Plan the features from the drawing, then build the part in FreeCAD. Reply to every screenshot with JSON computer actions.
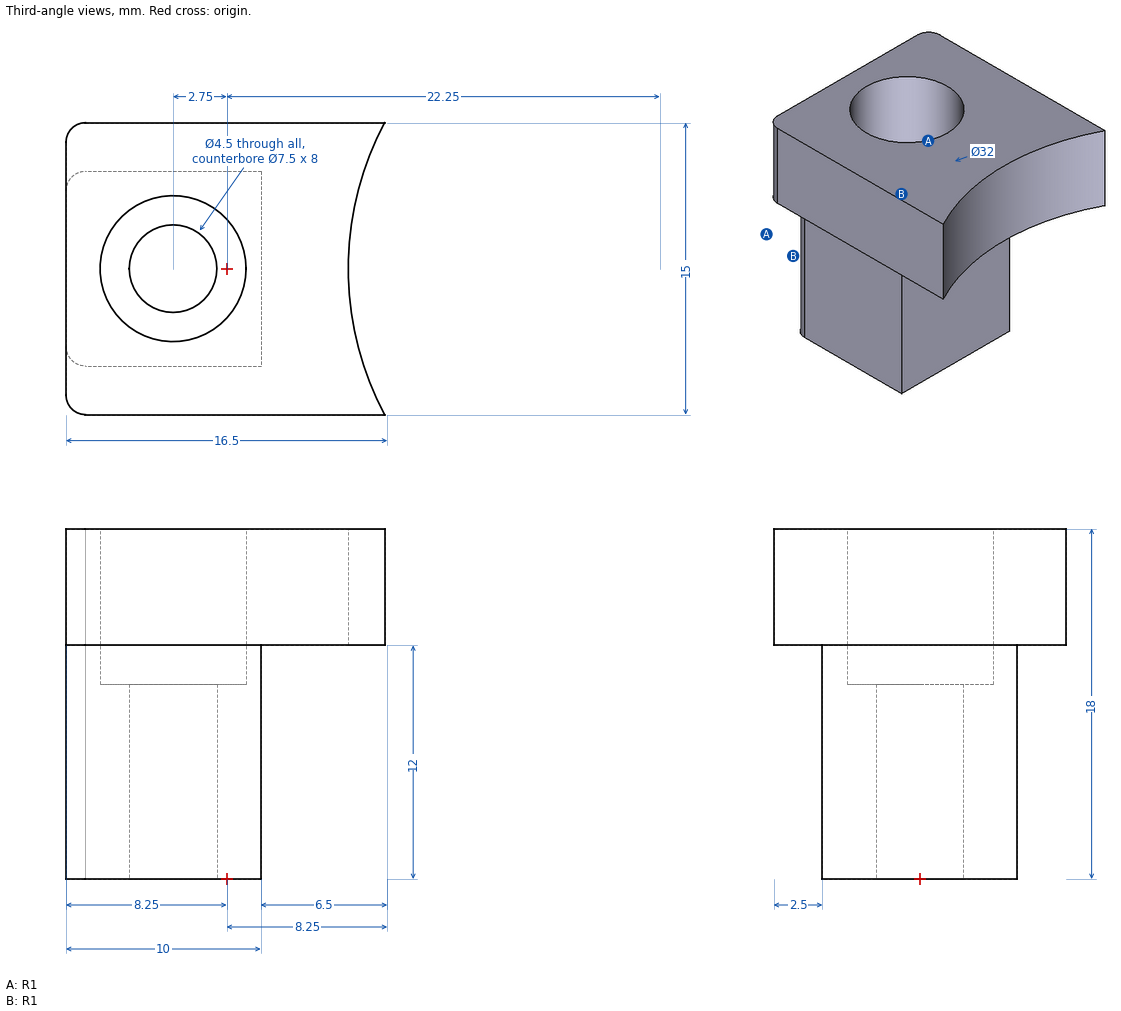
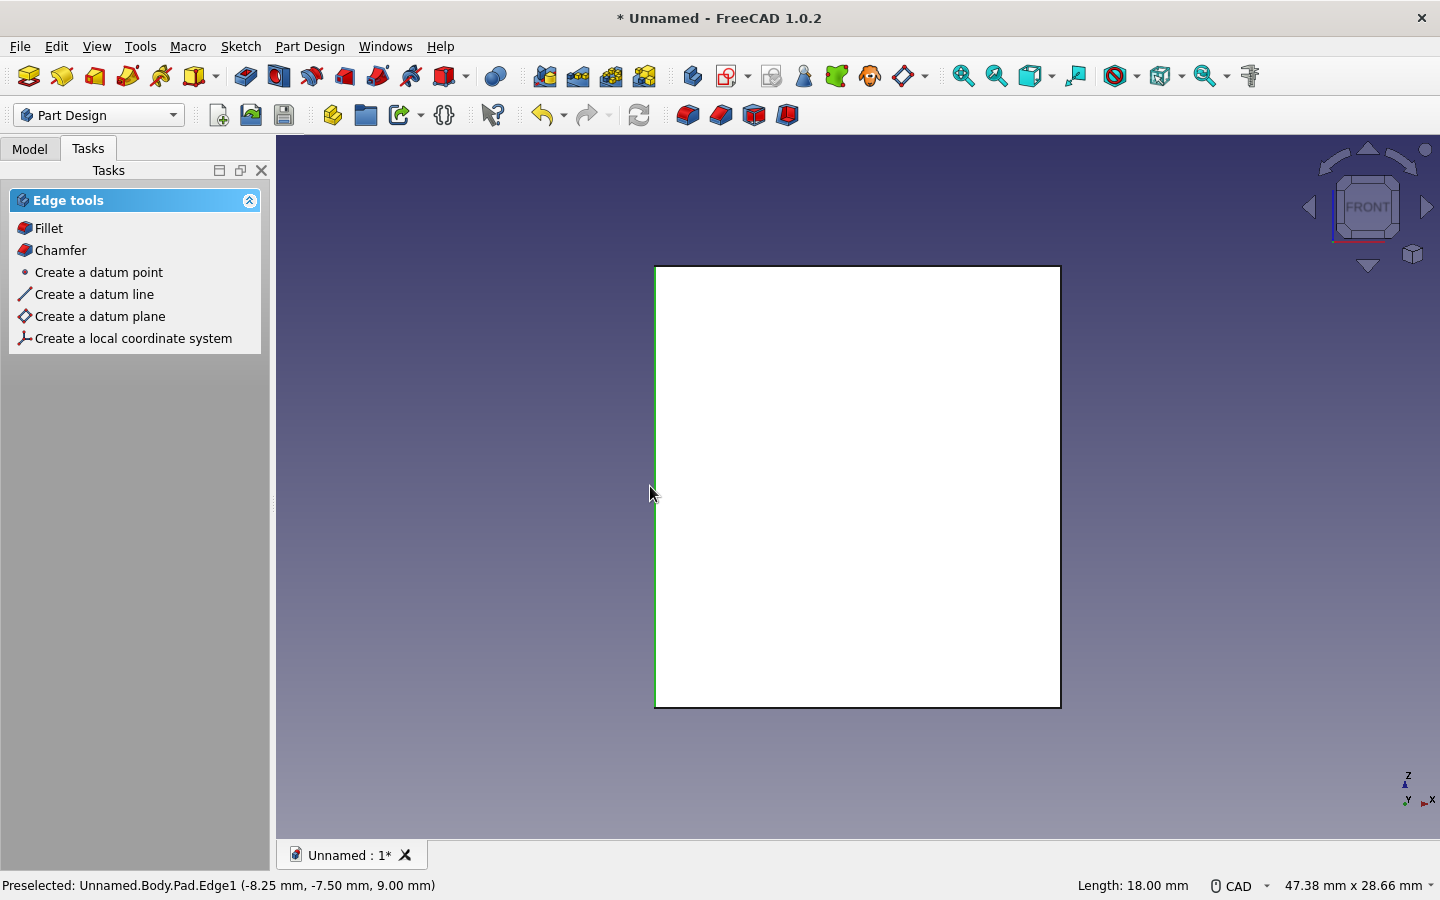
{"action": "key", "text": "3"}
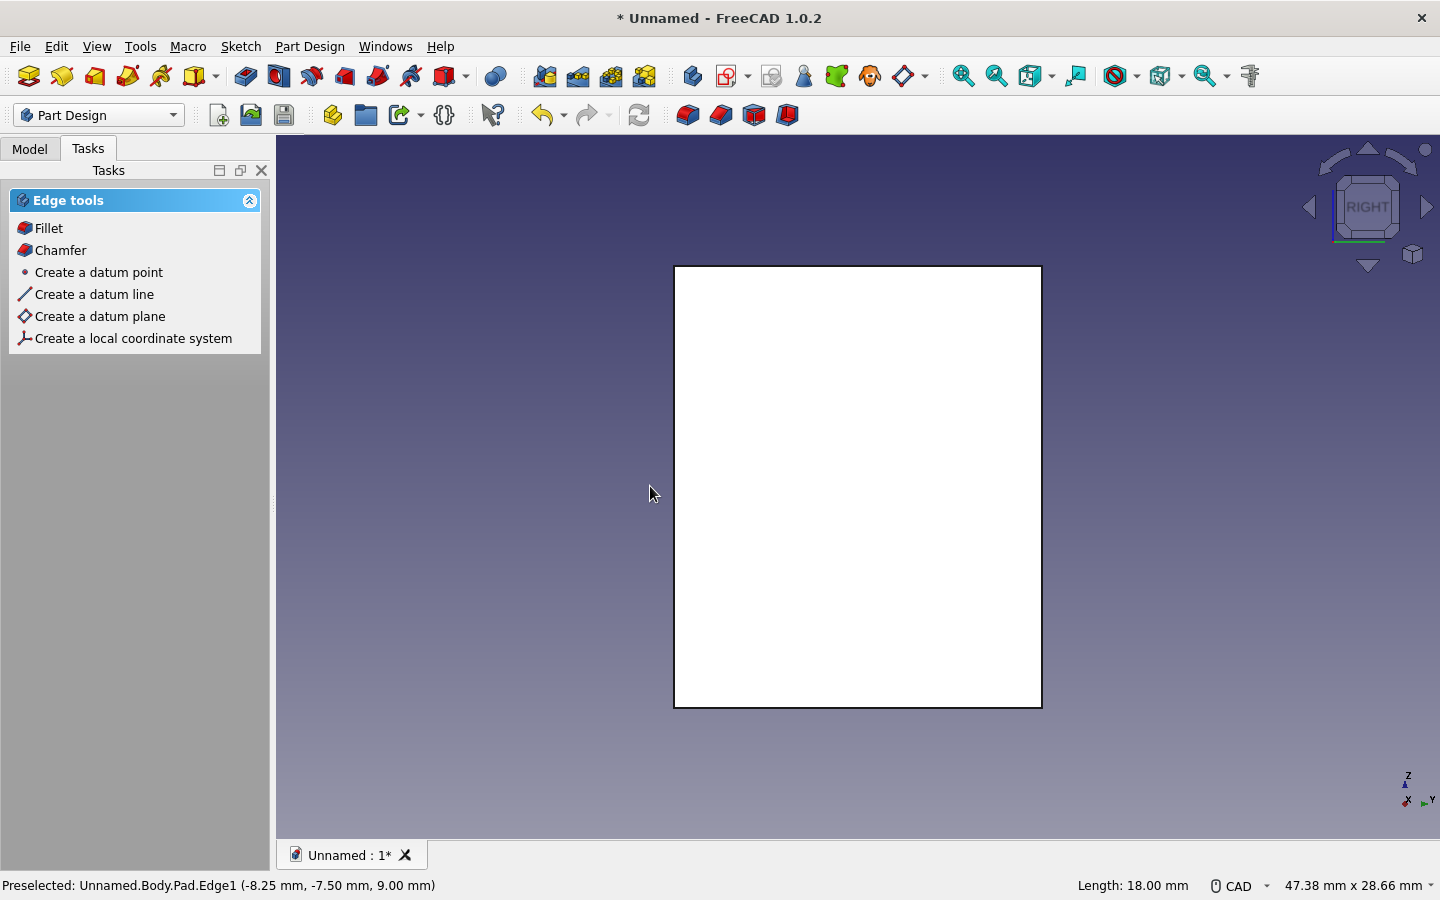
{"action": "key", "text": "5"}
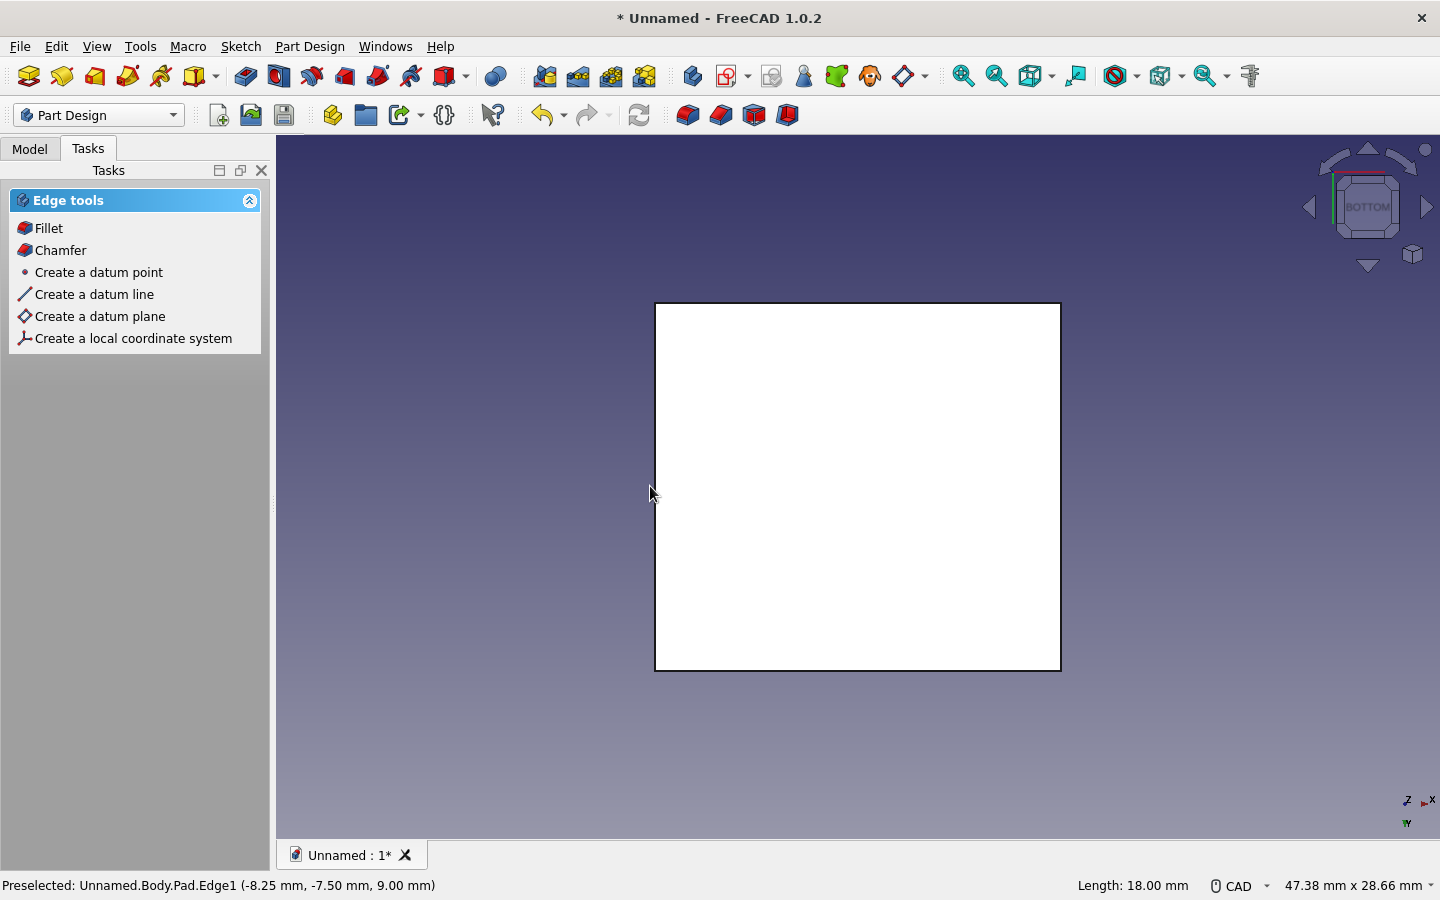
{"action": "key", "text": "4"}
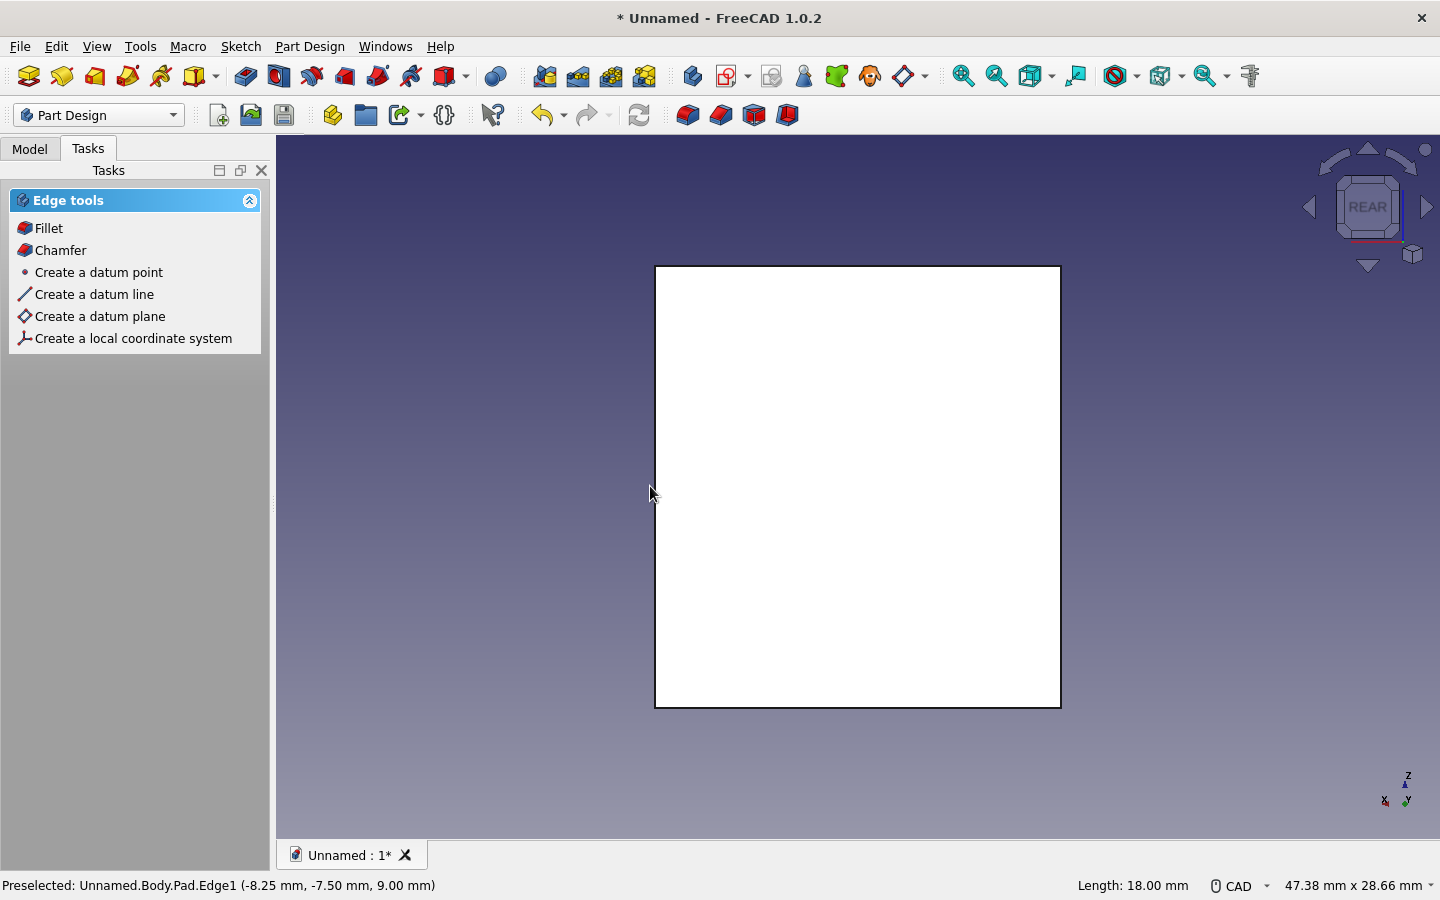
{"action": "left_click", "coordinate": [1061, 486], "text": "ctrl"}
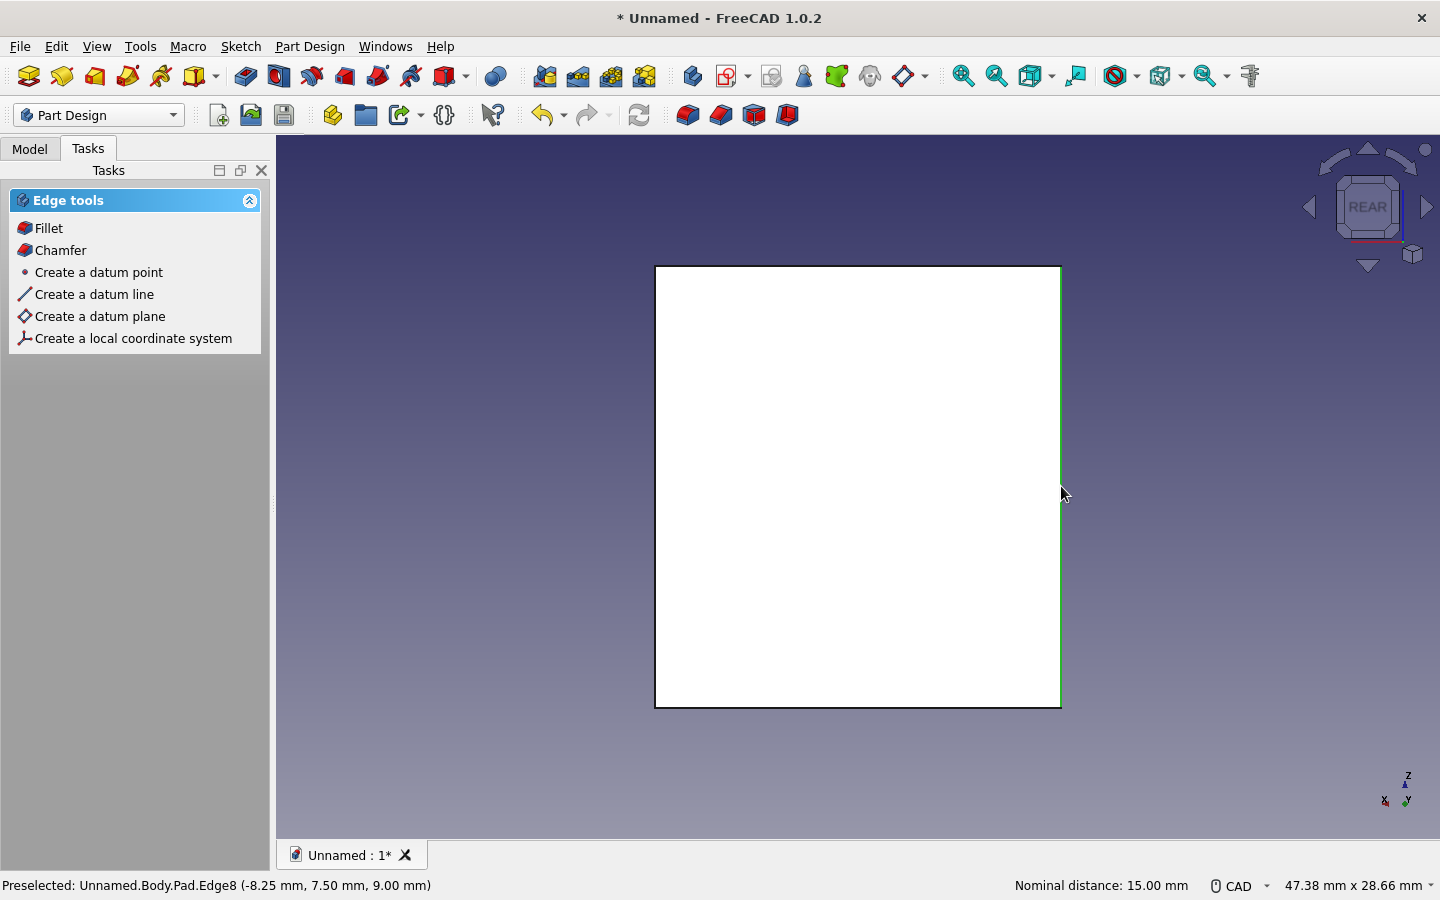
{"action": "left_click", "coordinate": [688, 116]}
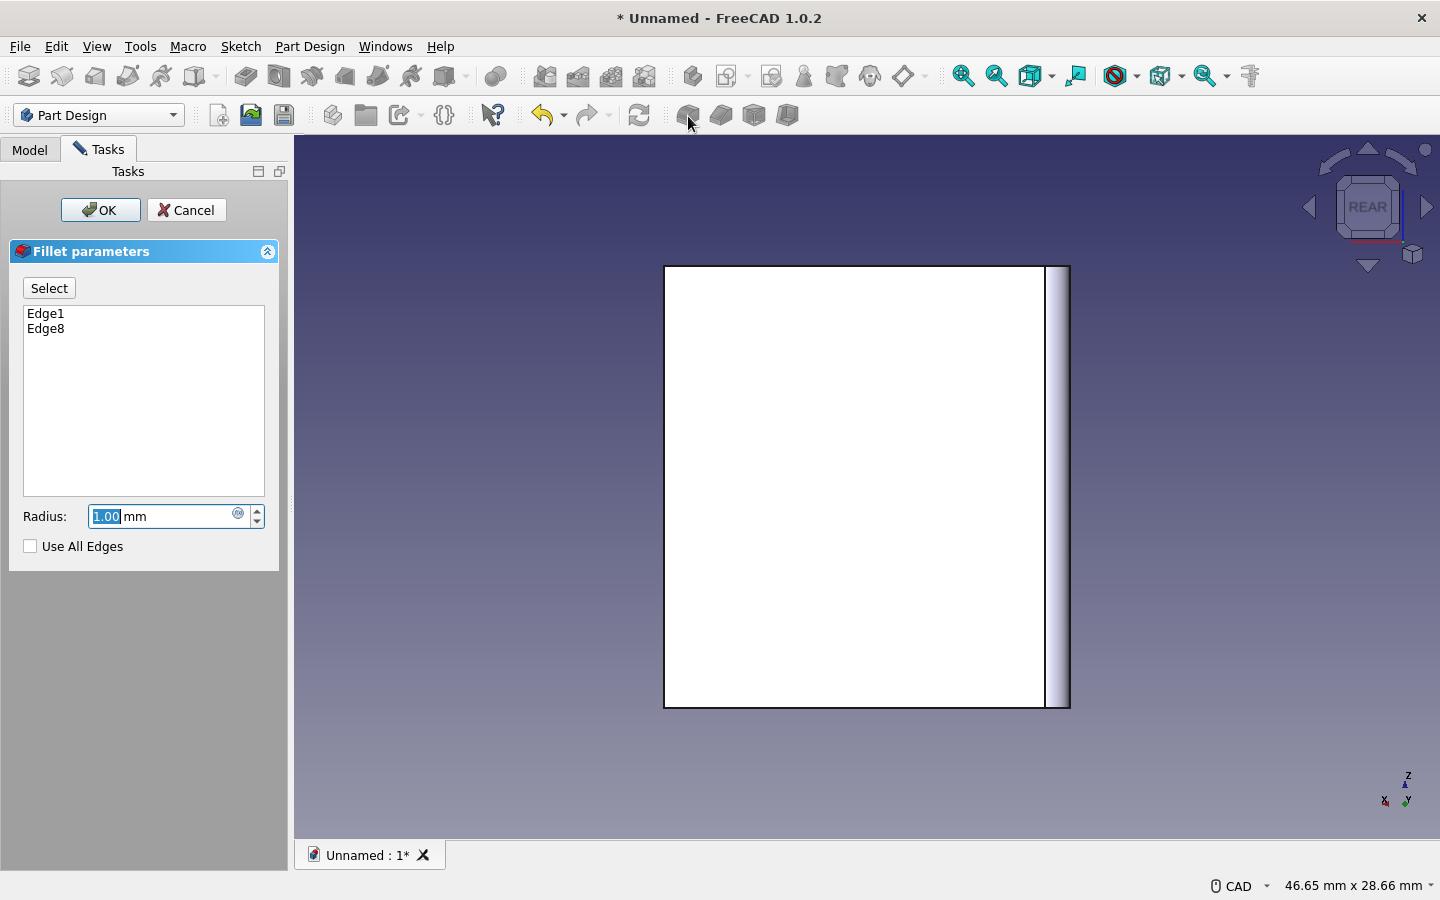
{"action": "type", "text": "1"}
{"action": "key", "text": "Tab"}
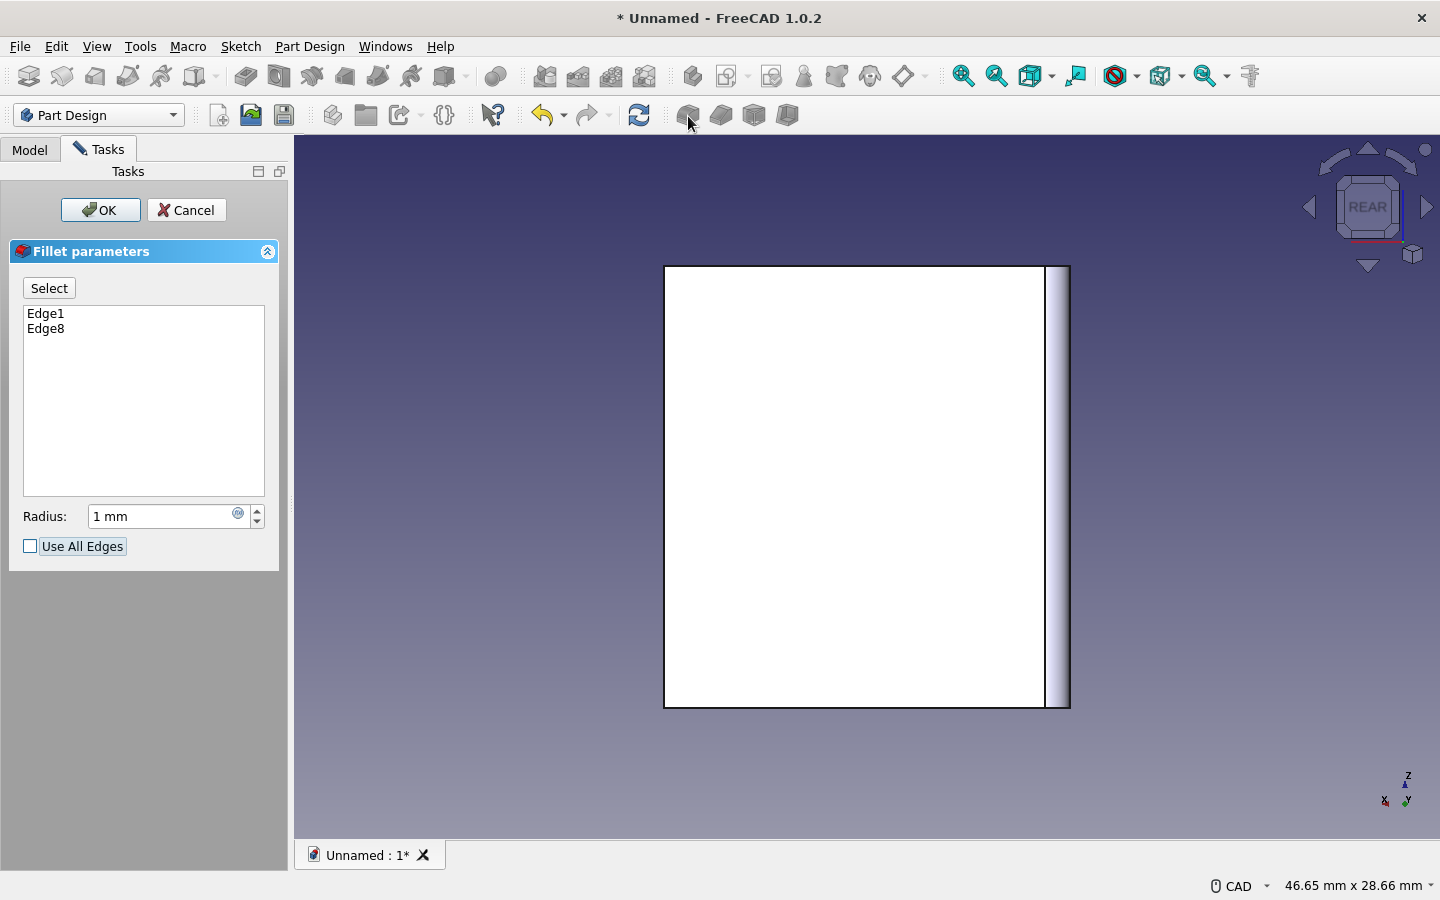
{"action": "left_click", "coordinate": [101, 210]}